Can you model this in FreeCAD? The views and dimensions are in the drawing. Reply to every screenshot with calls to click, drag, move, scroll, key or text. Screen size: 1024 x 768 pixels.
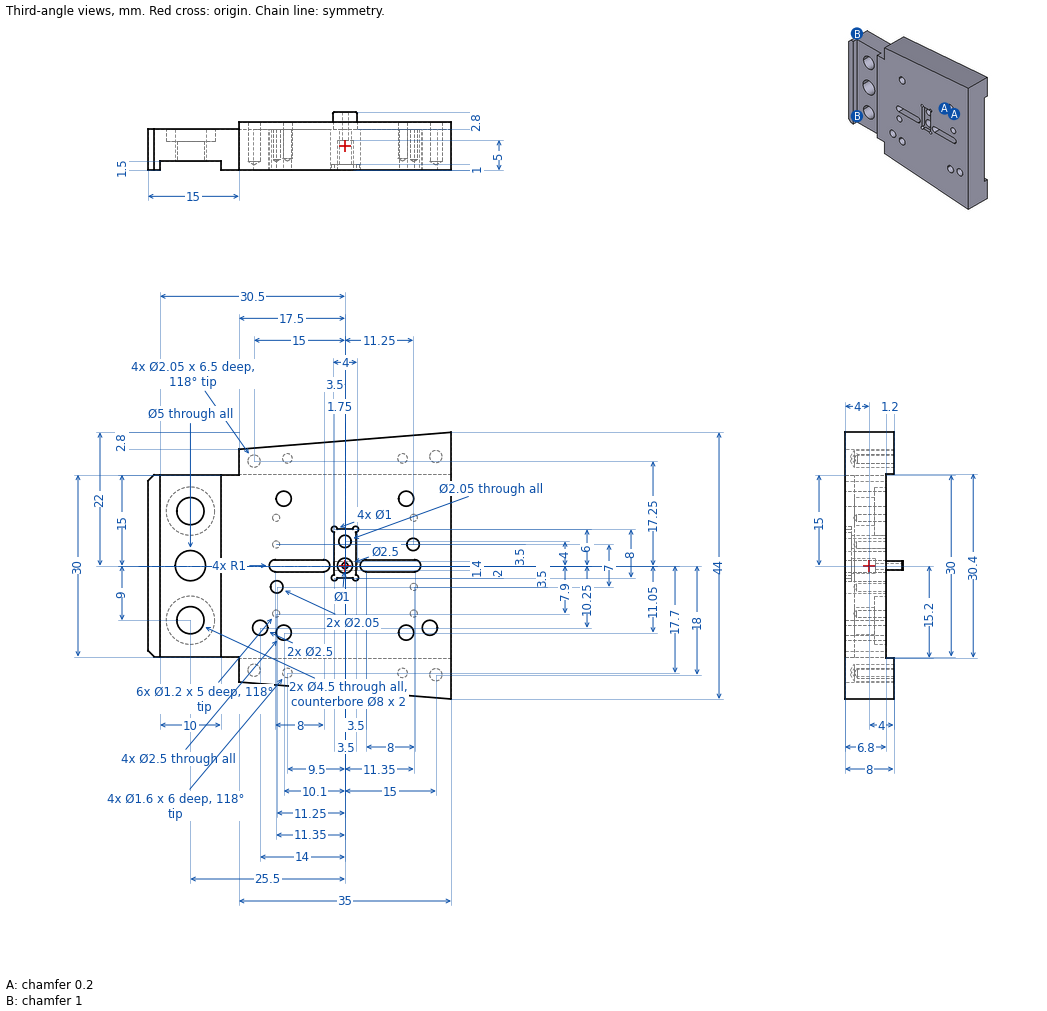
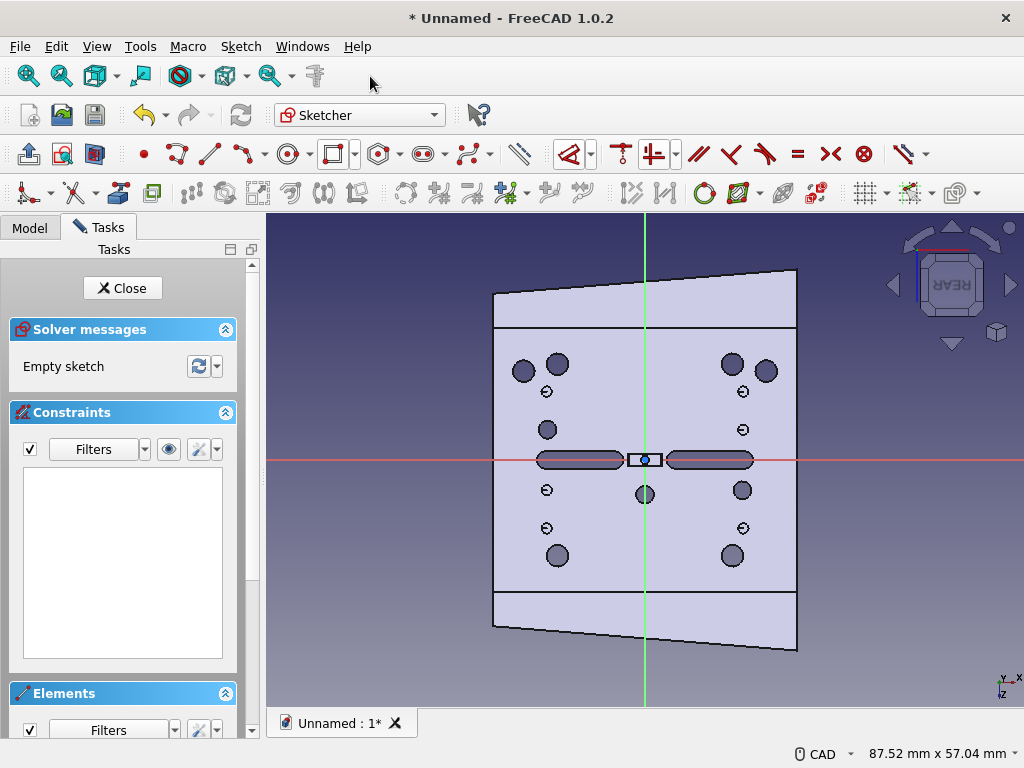
click(288, 154)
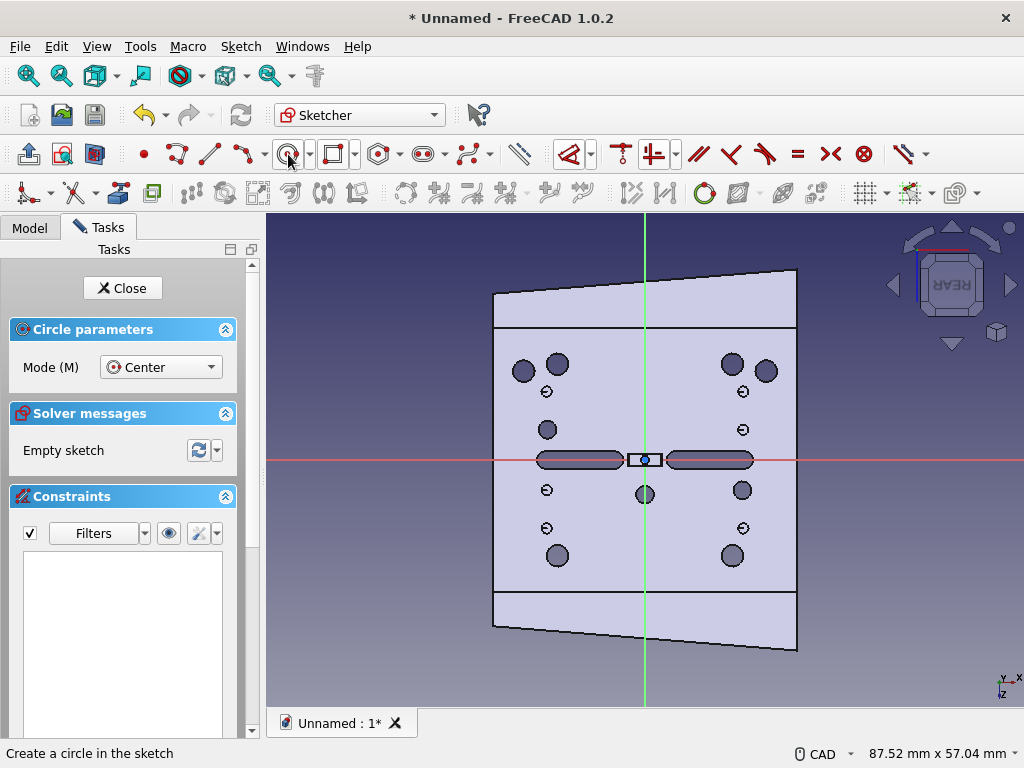
scroll(515, 609, up, 5)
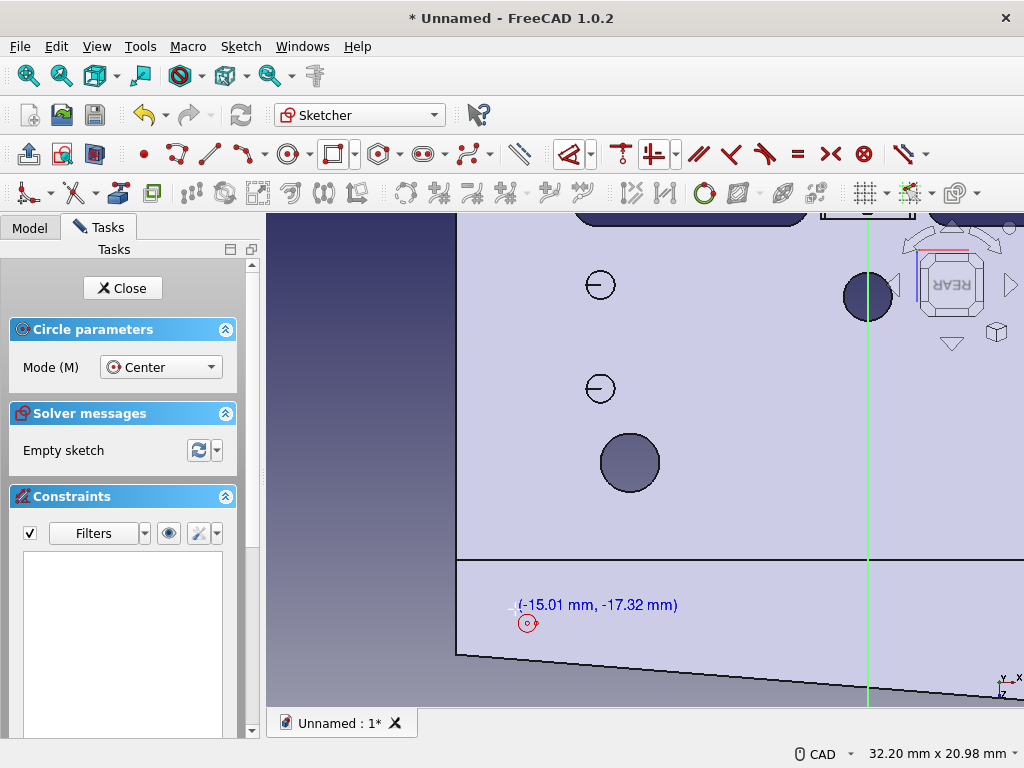
click(515, 609)
move(532, 592)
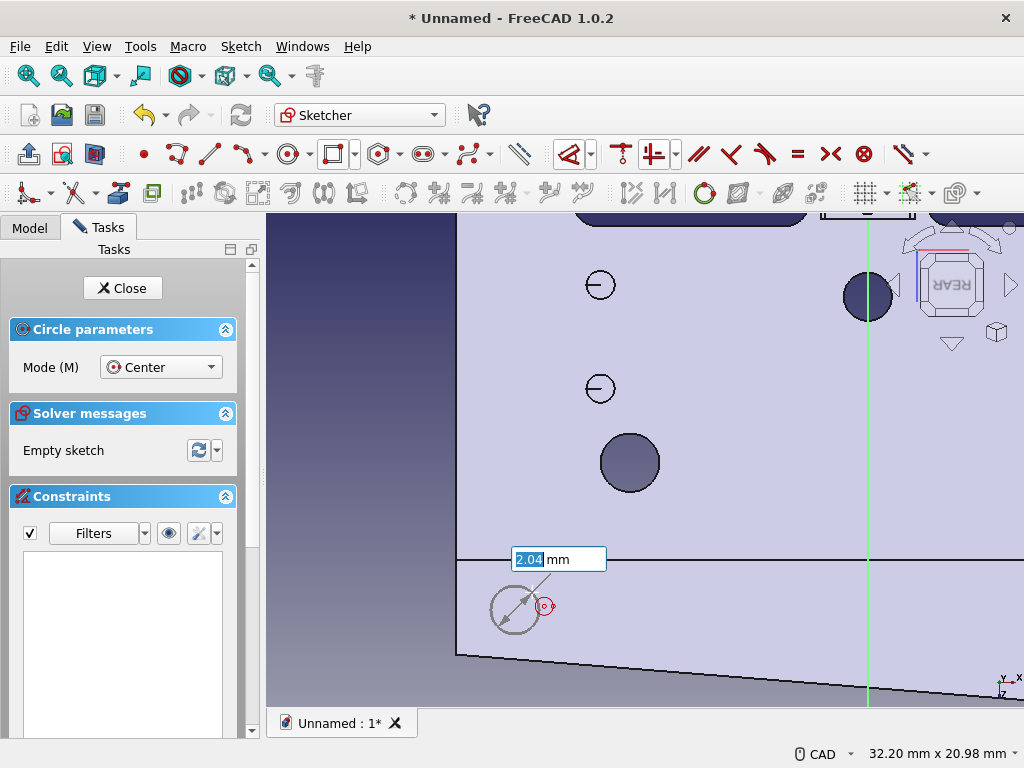
text(2.05)
key(Return)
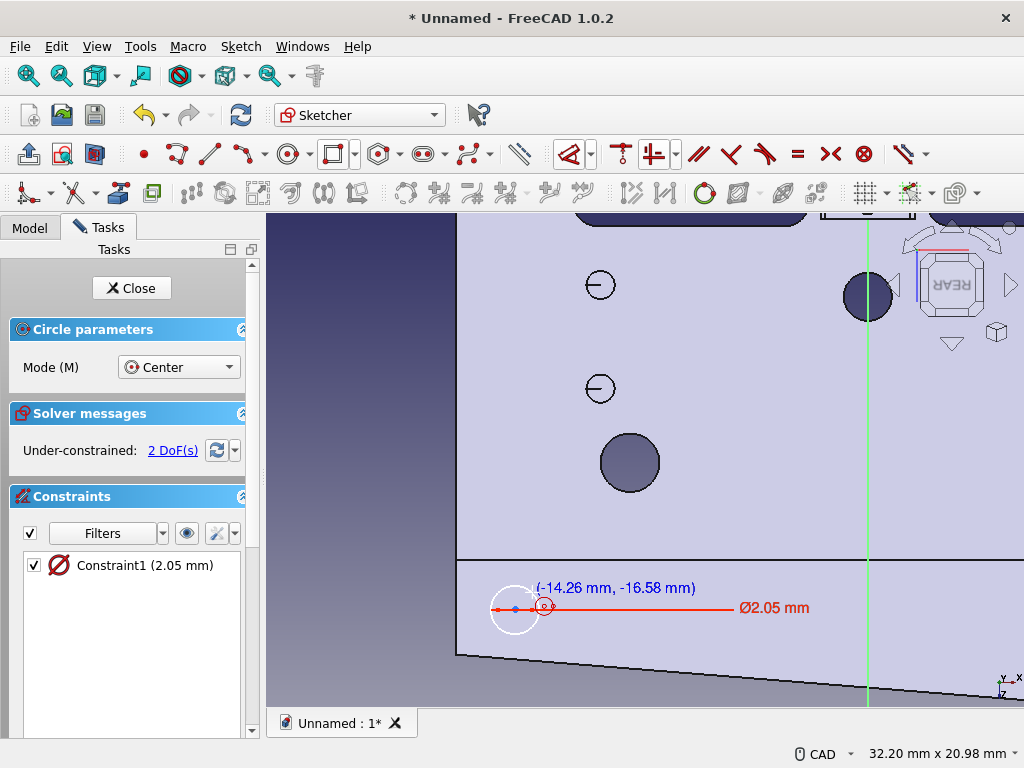
scroll(407, 610, down, 5)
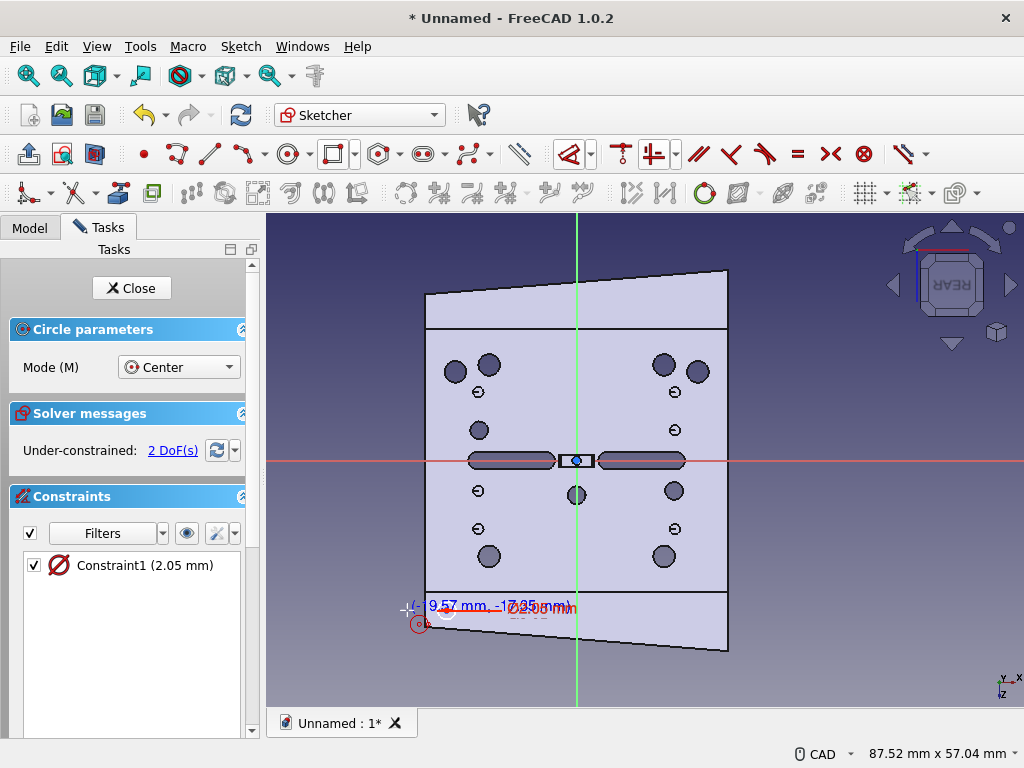
scroll(447, 311, up, 5)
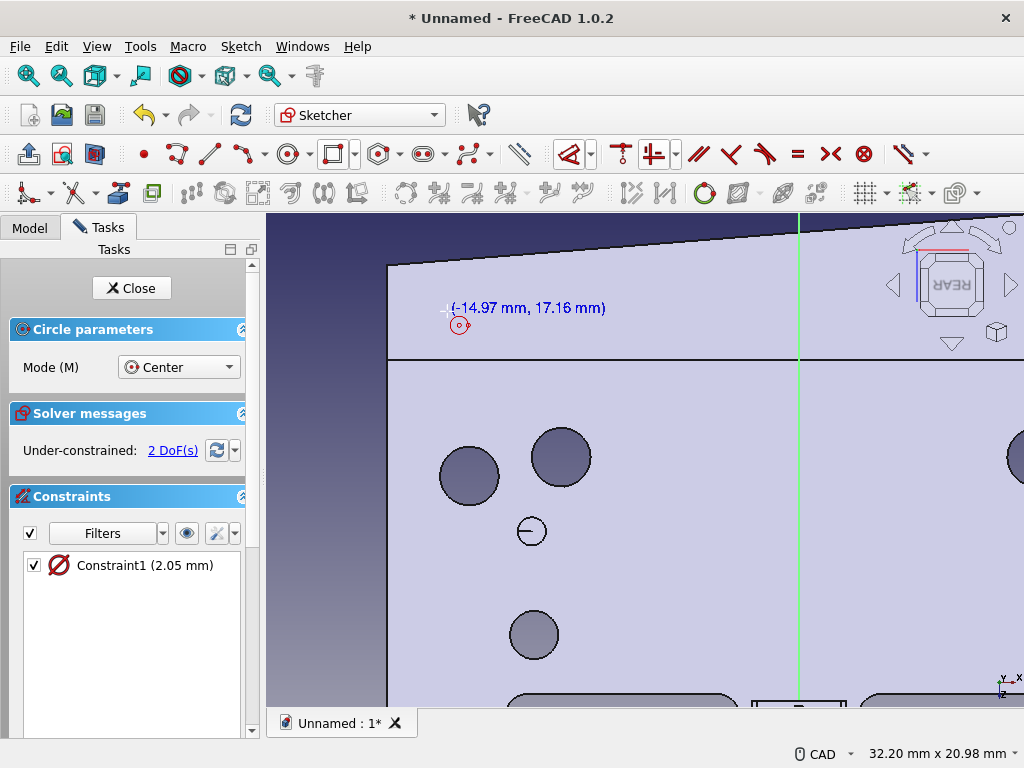
click(446, 311)
move(463, 294)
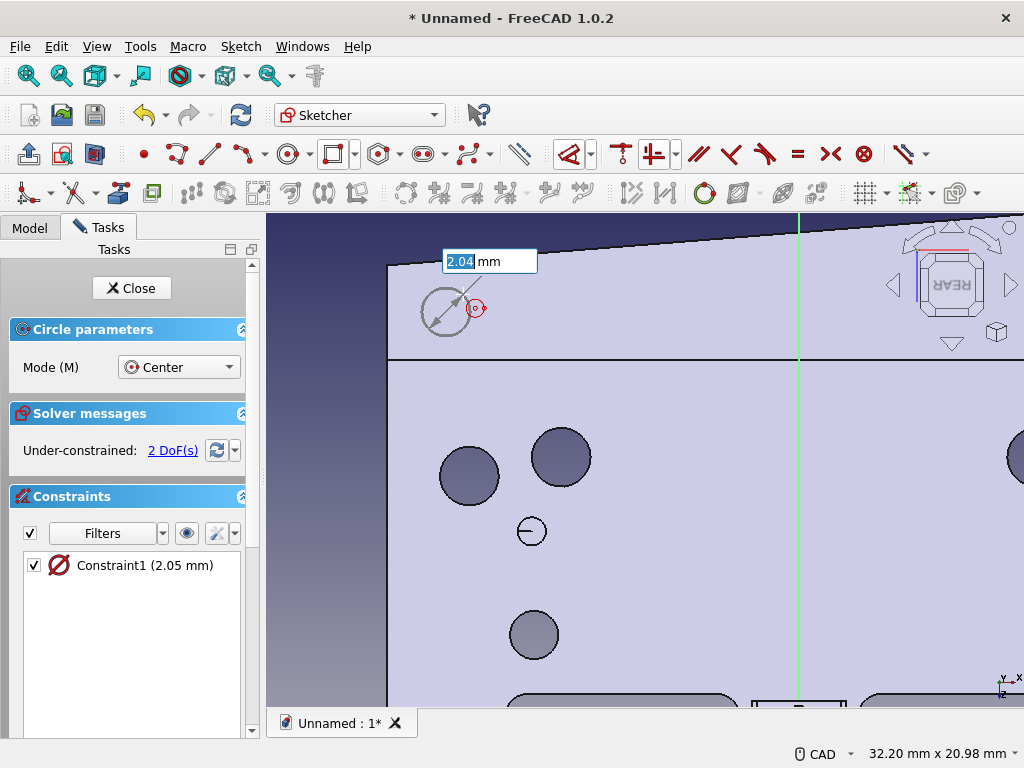
text(2.05)
key(Return)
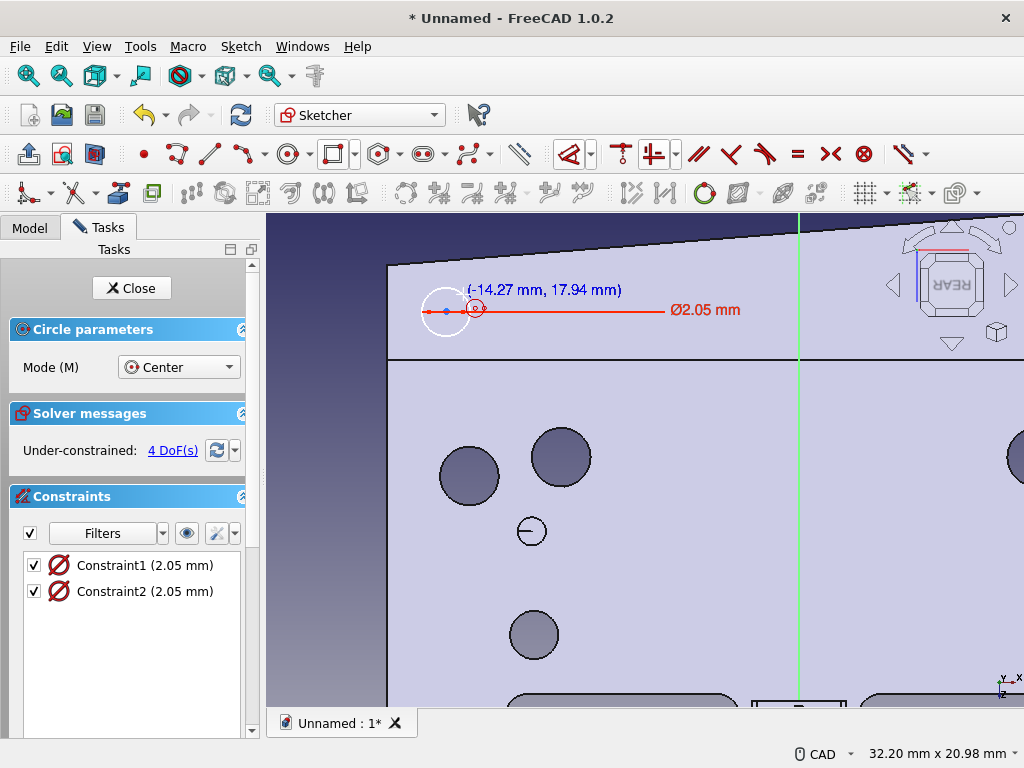
scroll(447, 310, down, 5)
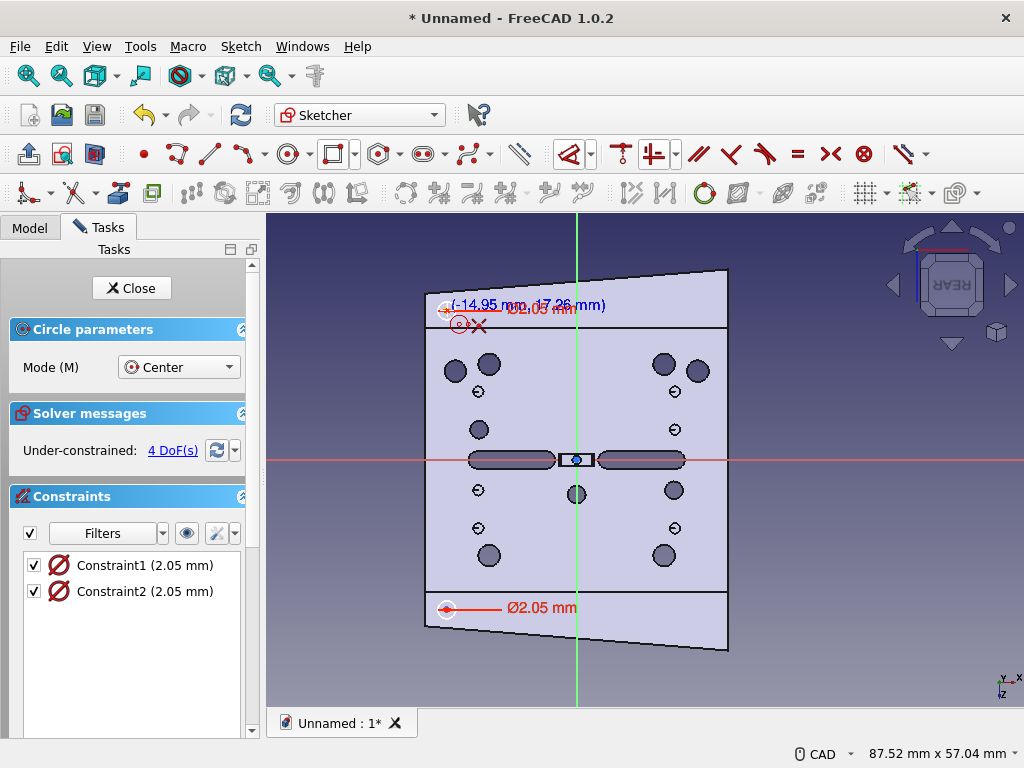
scroll(707, 304, up, 5)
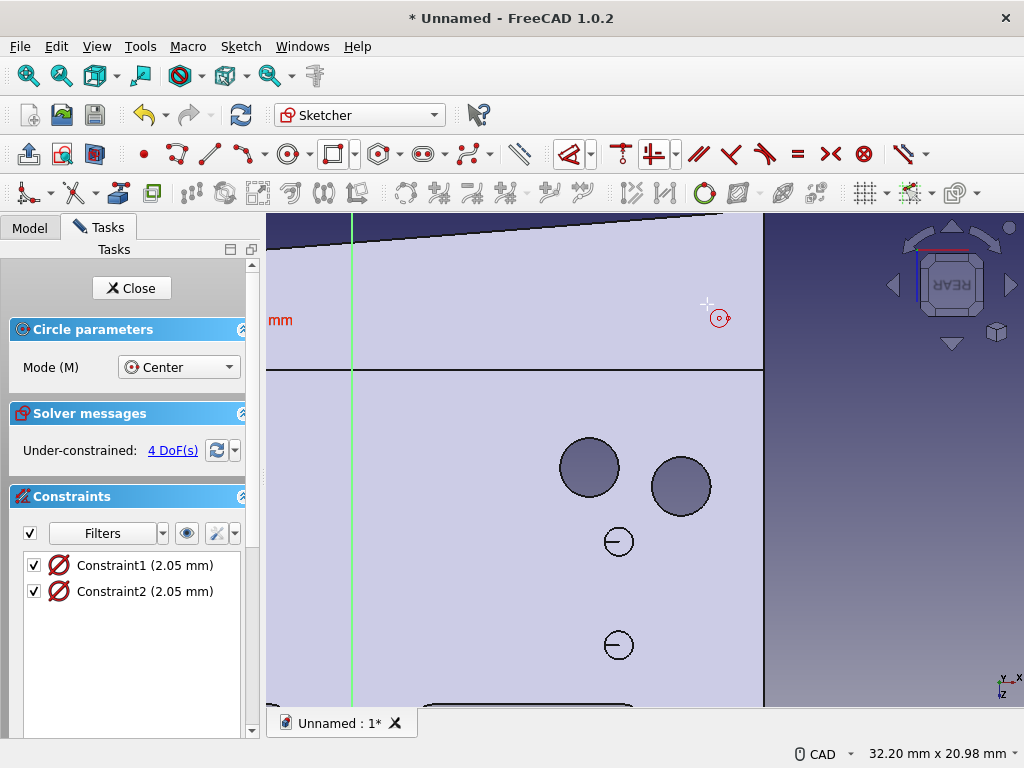
click(705, 304)
move(722, 287)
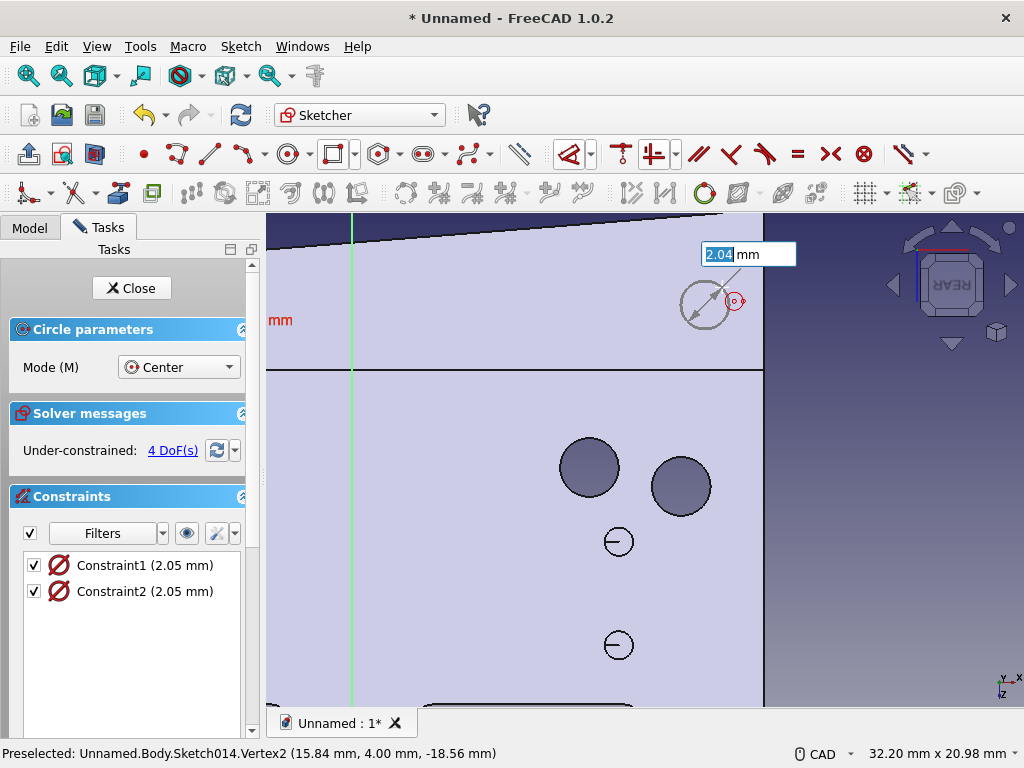
text(2.05)
key(Return)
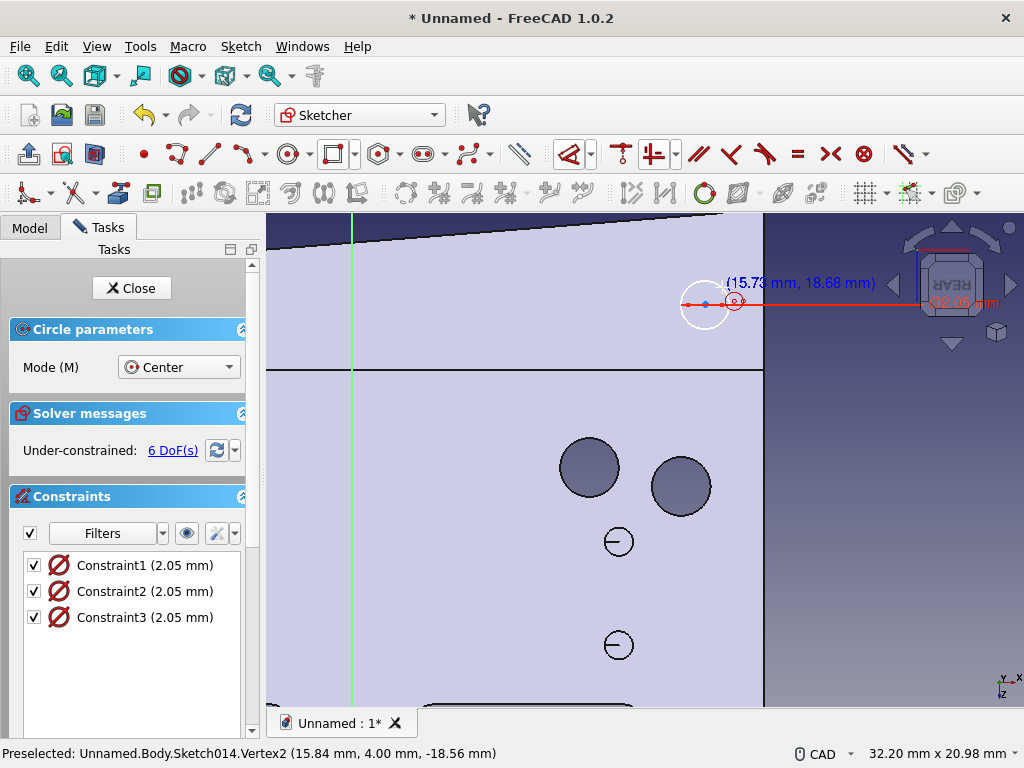
scroll(707, 304, down, 5)